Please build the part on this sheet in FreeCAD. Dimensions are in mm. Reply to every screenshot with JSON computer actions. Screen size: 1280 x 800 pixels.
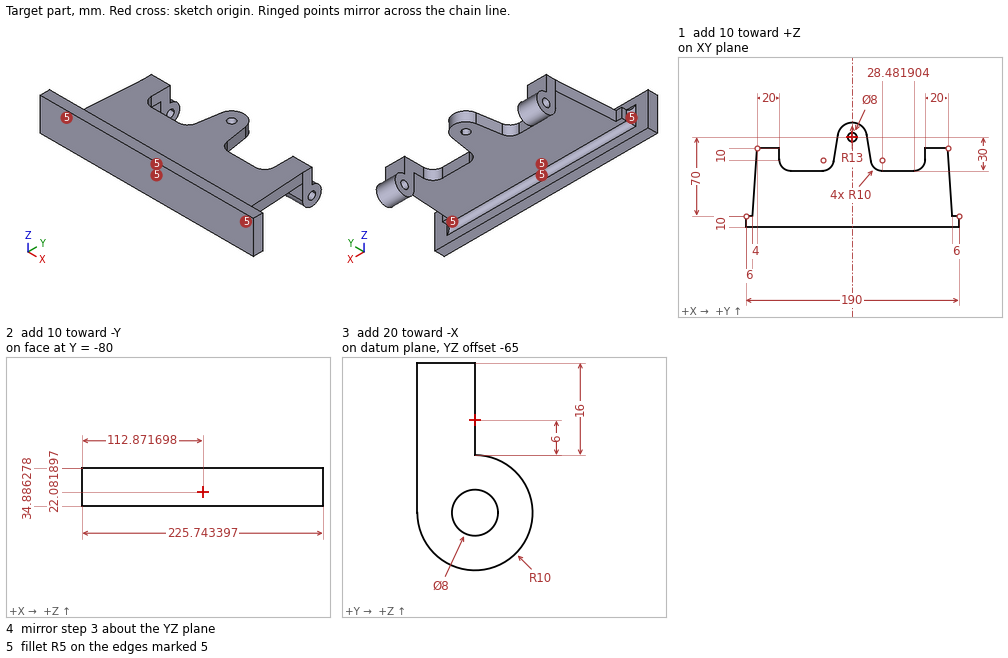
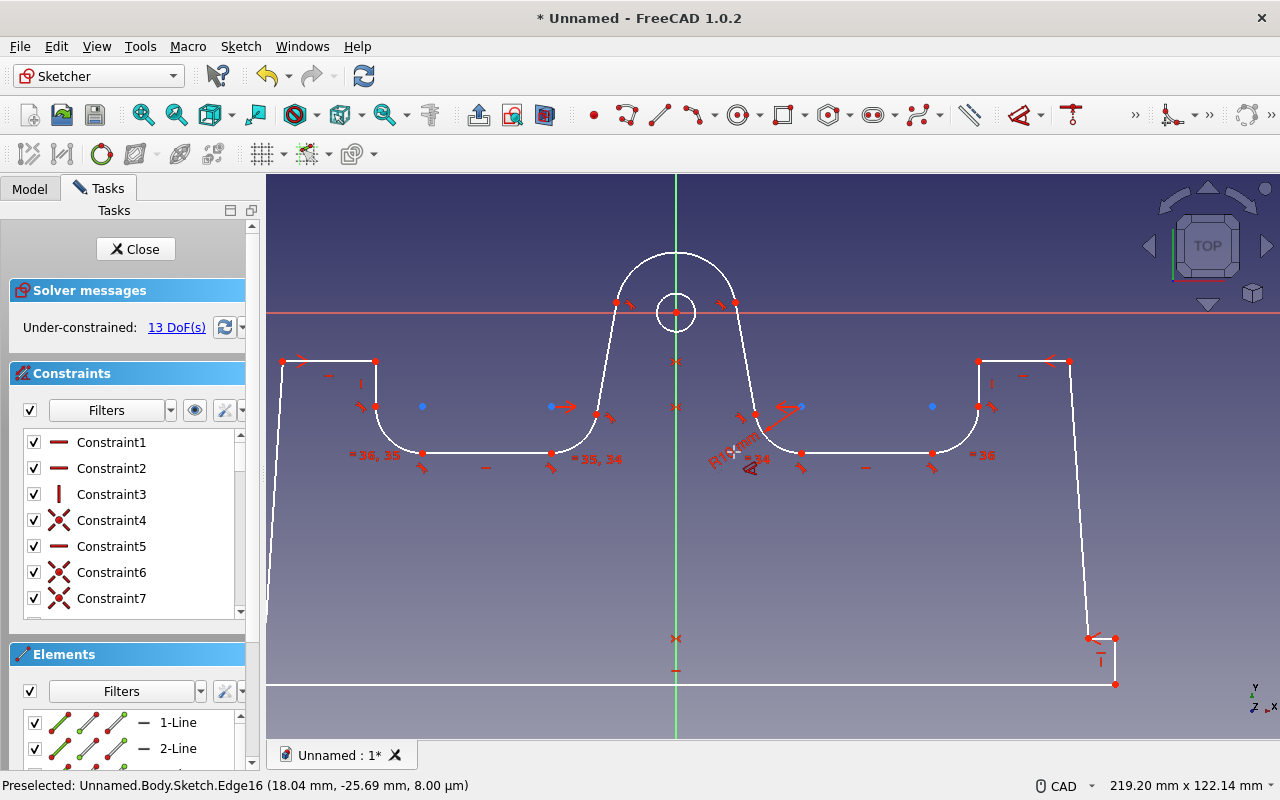
{"action": "left_click", "coordinate": [708, 262]}
{"action": "left_click", "coordinate": [725, 235]}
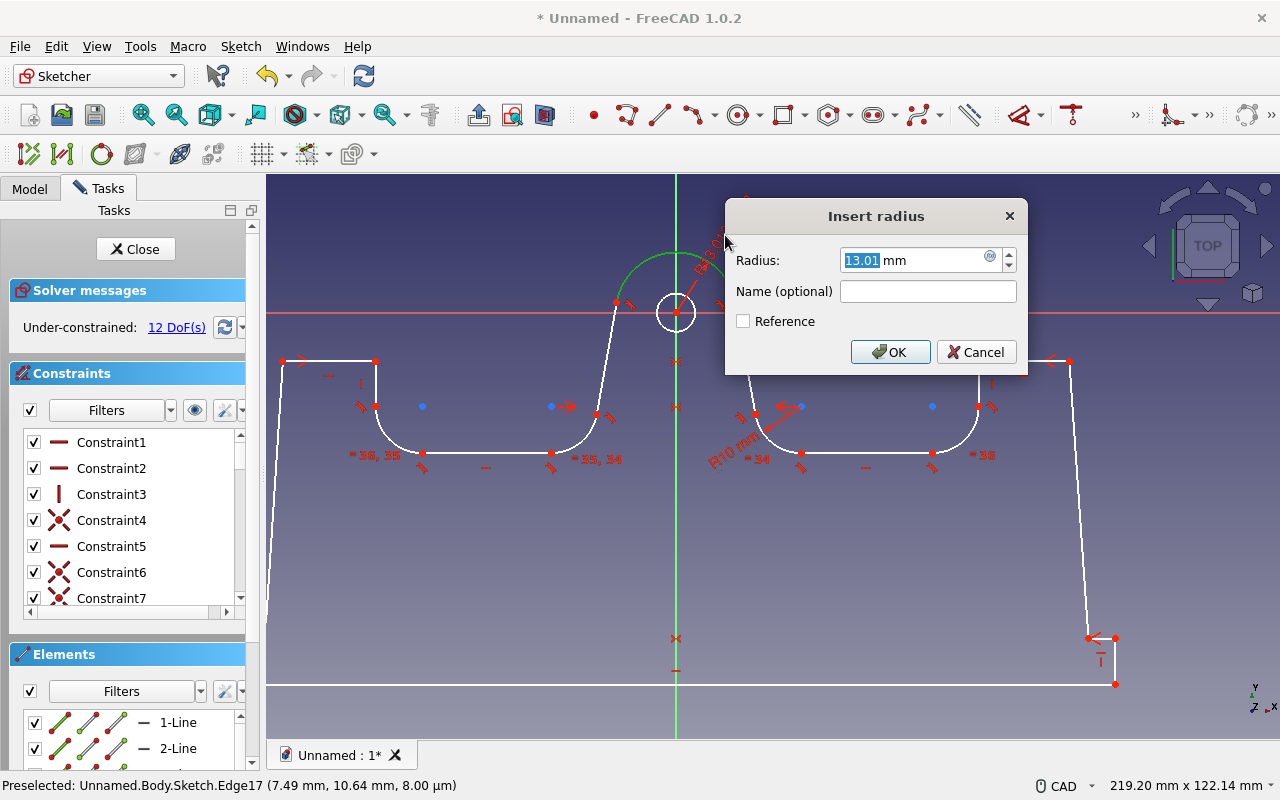
{"action": "type", "text": "13"}
{"action": "key", "text": "Return"}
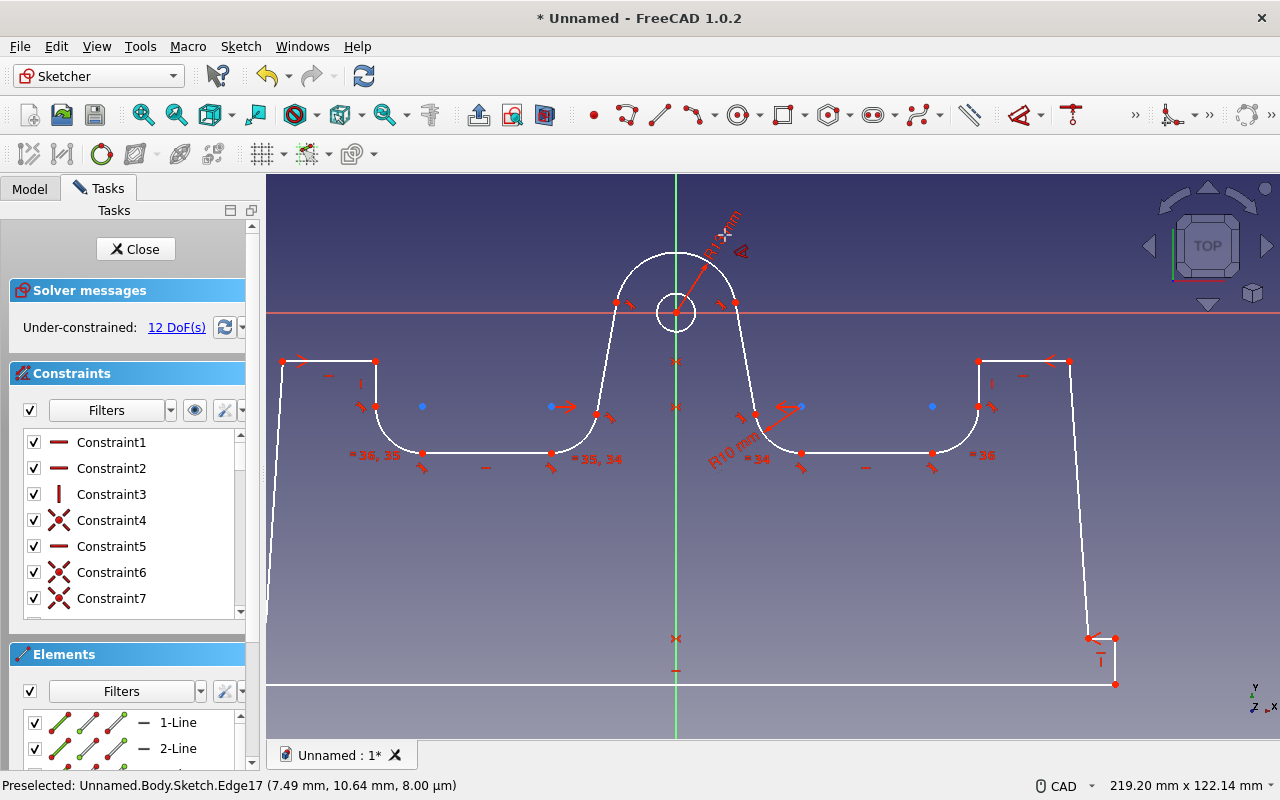
{"action": "left_click", "coordinate": [690, 299]}
{"action": "left_click", "coordinate": [712, 349]}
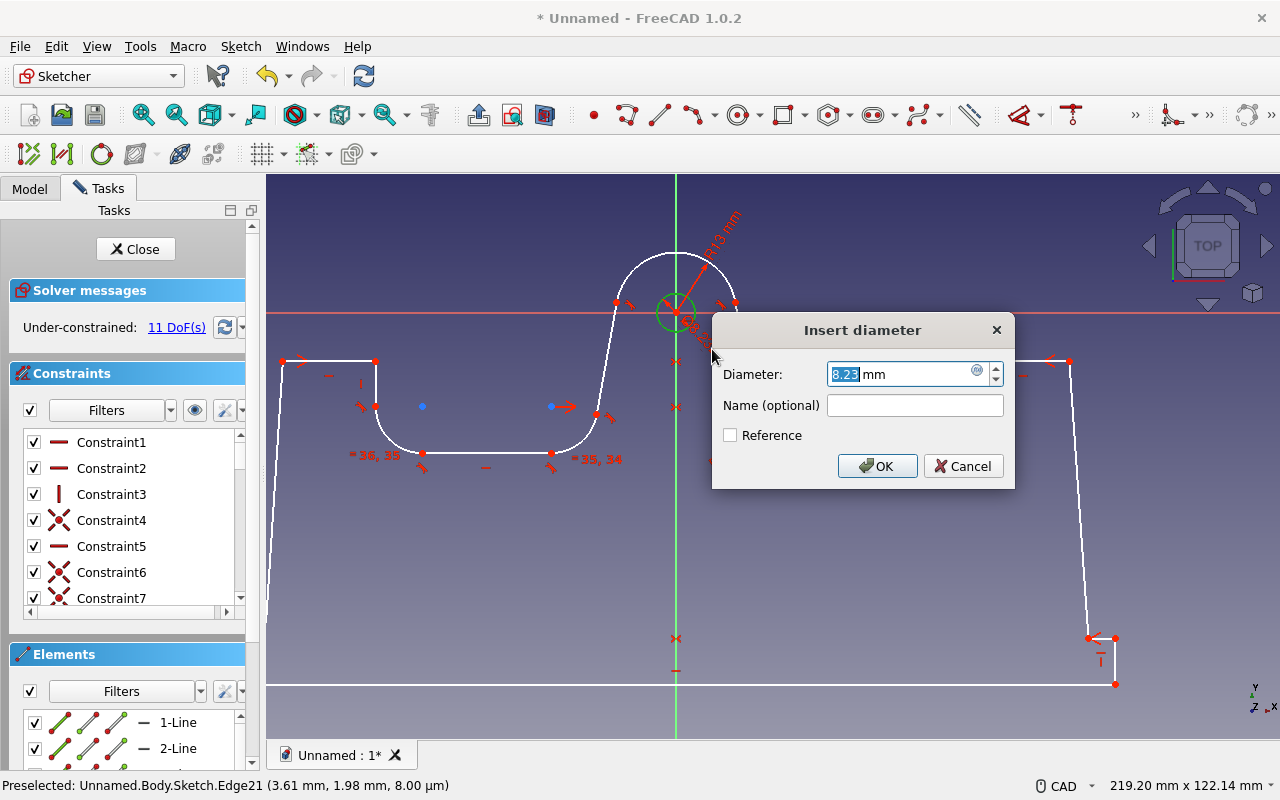
{"action": "type", "text": "8"}
{"action": "key", "text": "Return"}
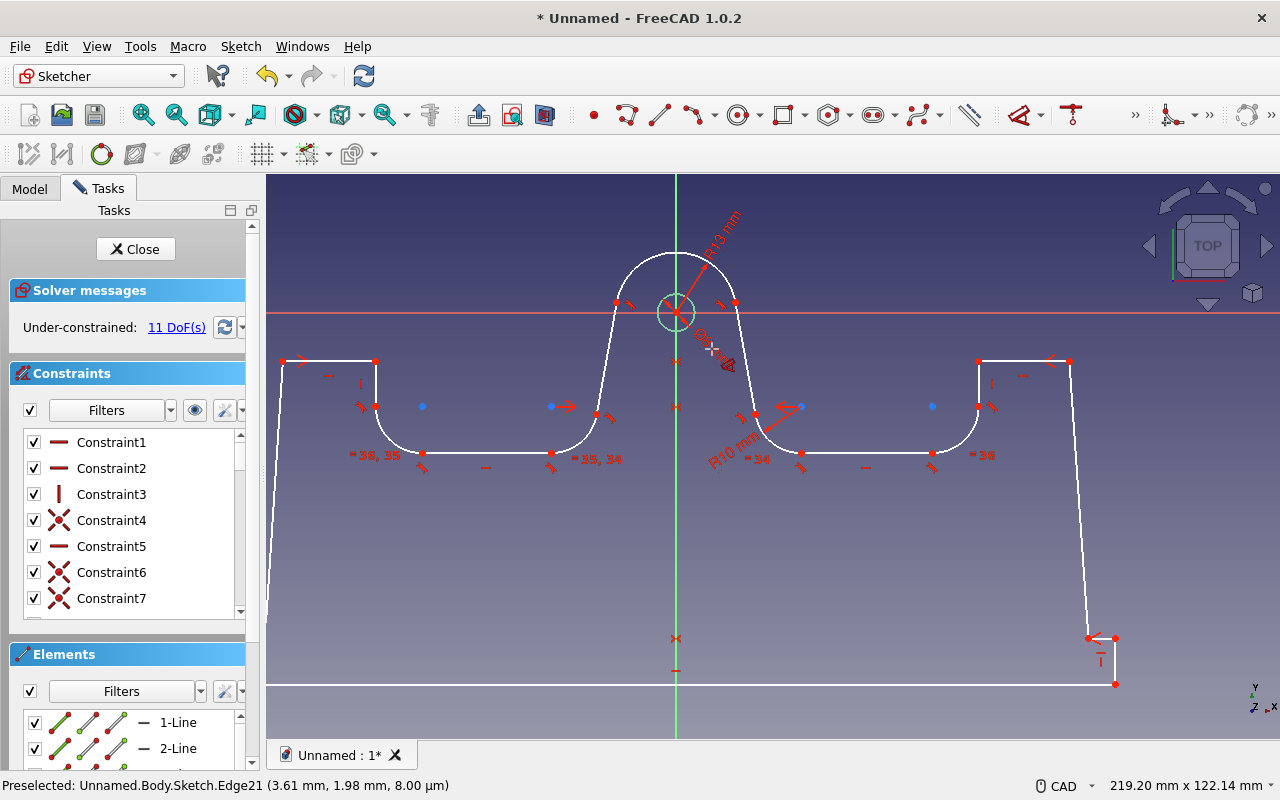
{"action": "scroll", "coordinate": [762, 434], "scroll_direction": "down", "scroll_amount": 2}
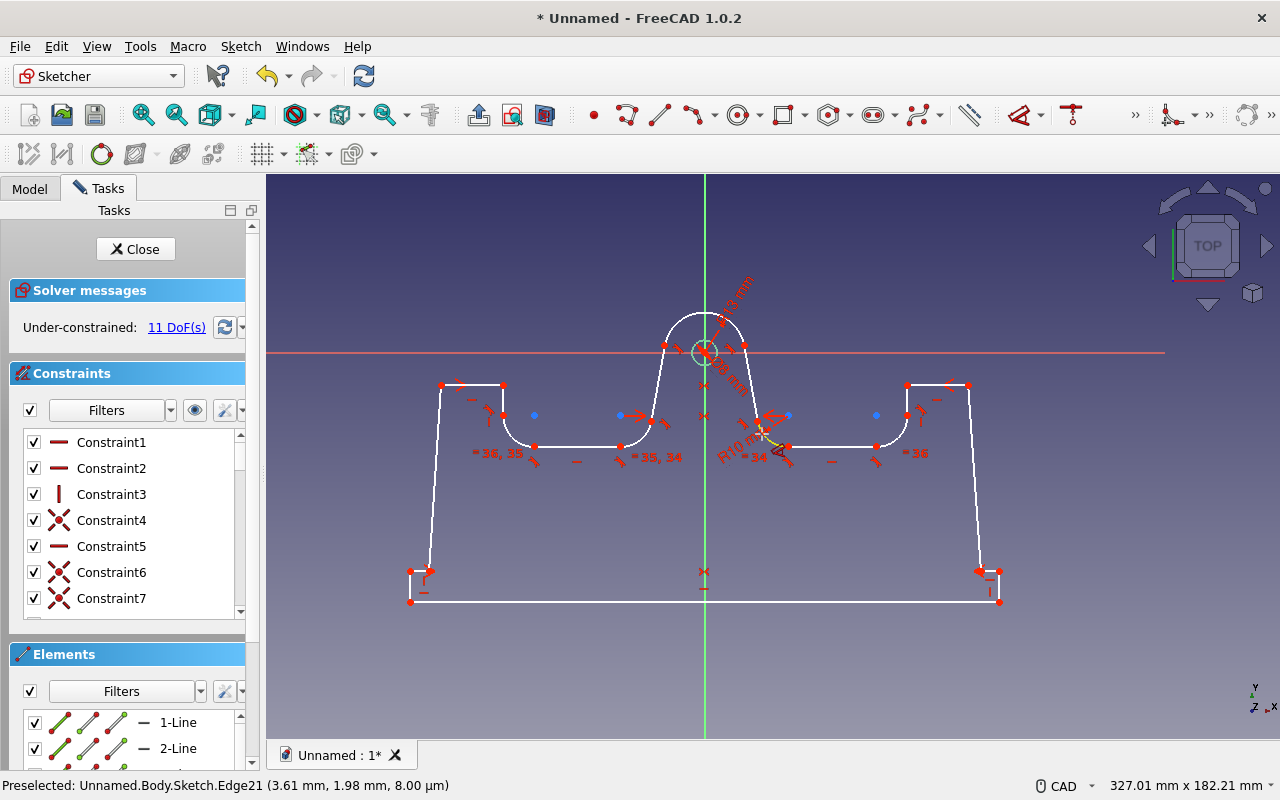
{"action": "scroll", "coordinate": [421, 571], "scroll_direction": "up", "scroll_amount": 4}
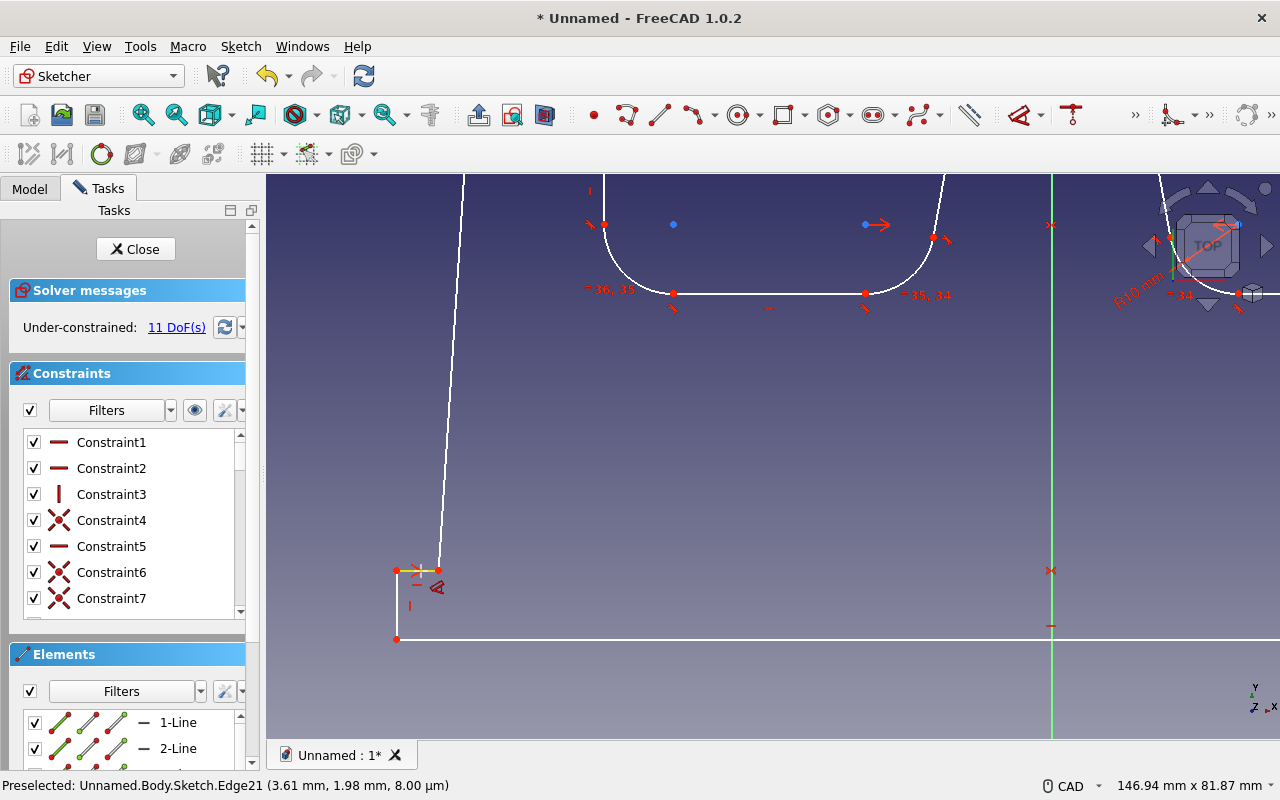
{"action": "left_click", "coordinate": [422, 571]}
{"action": "left_click", "coordinate": [418, 605]}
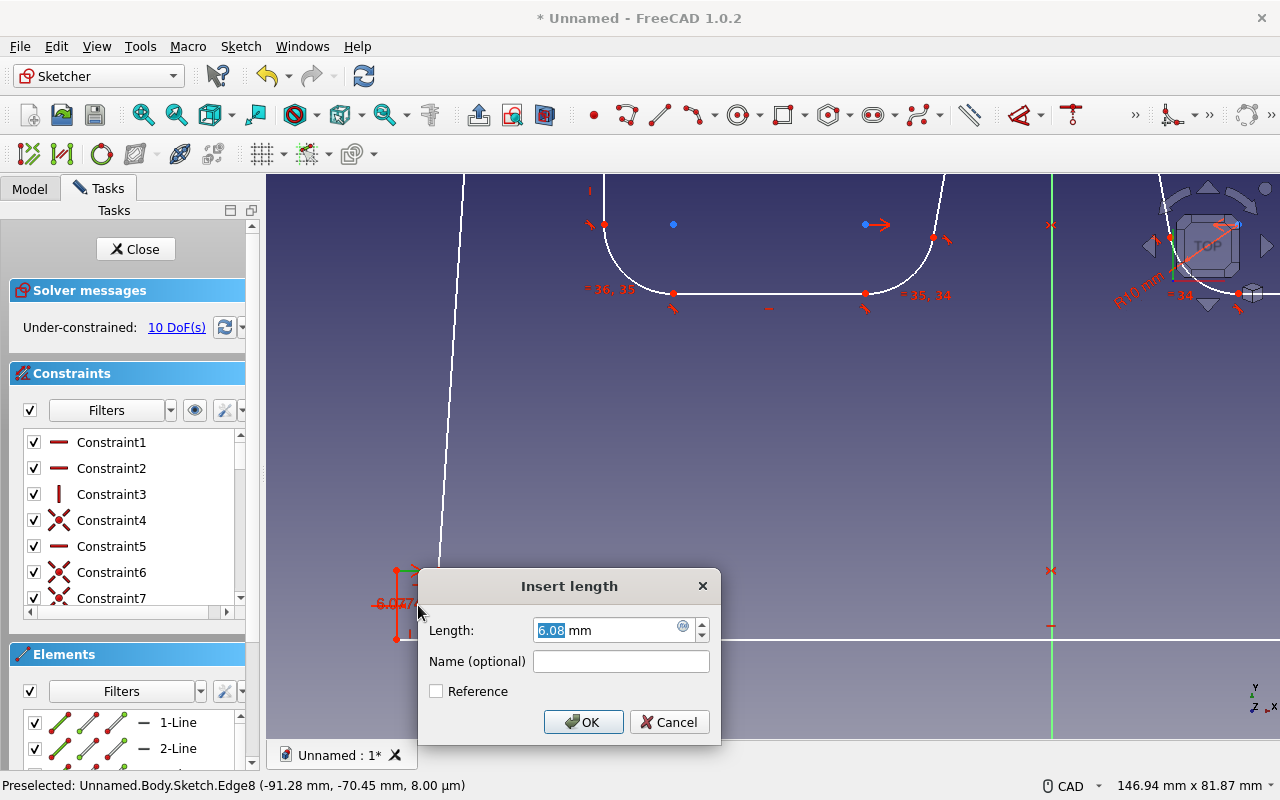
{"action": "type", "text": "6"}
{"action": "key", "text": "Return"}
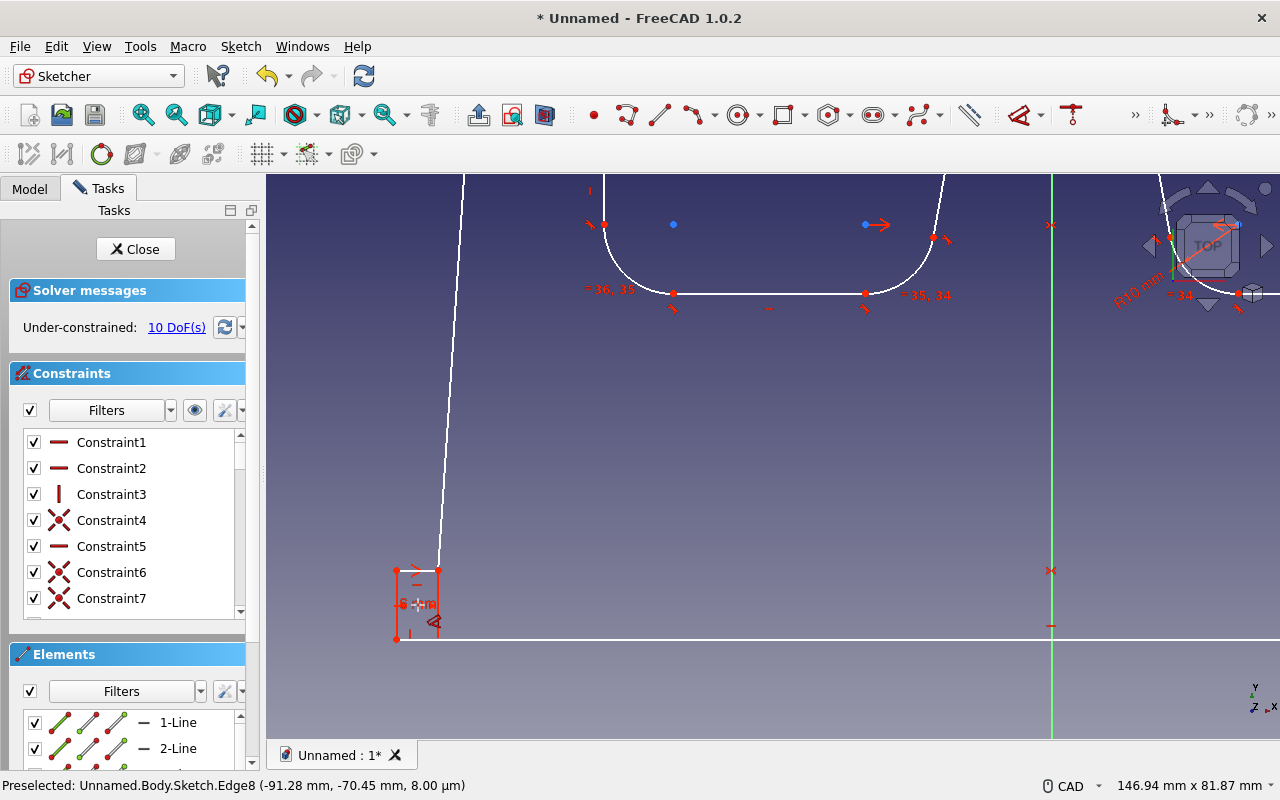
{"action": "scroll", "coordinate": [421, 571], "scroll_direction": "down", "scroll_amount": 4}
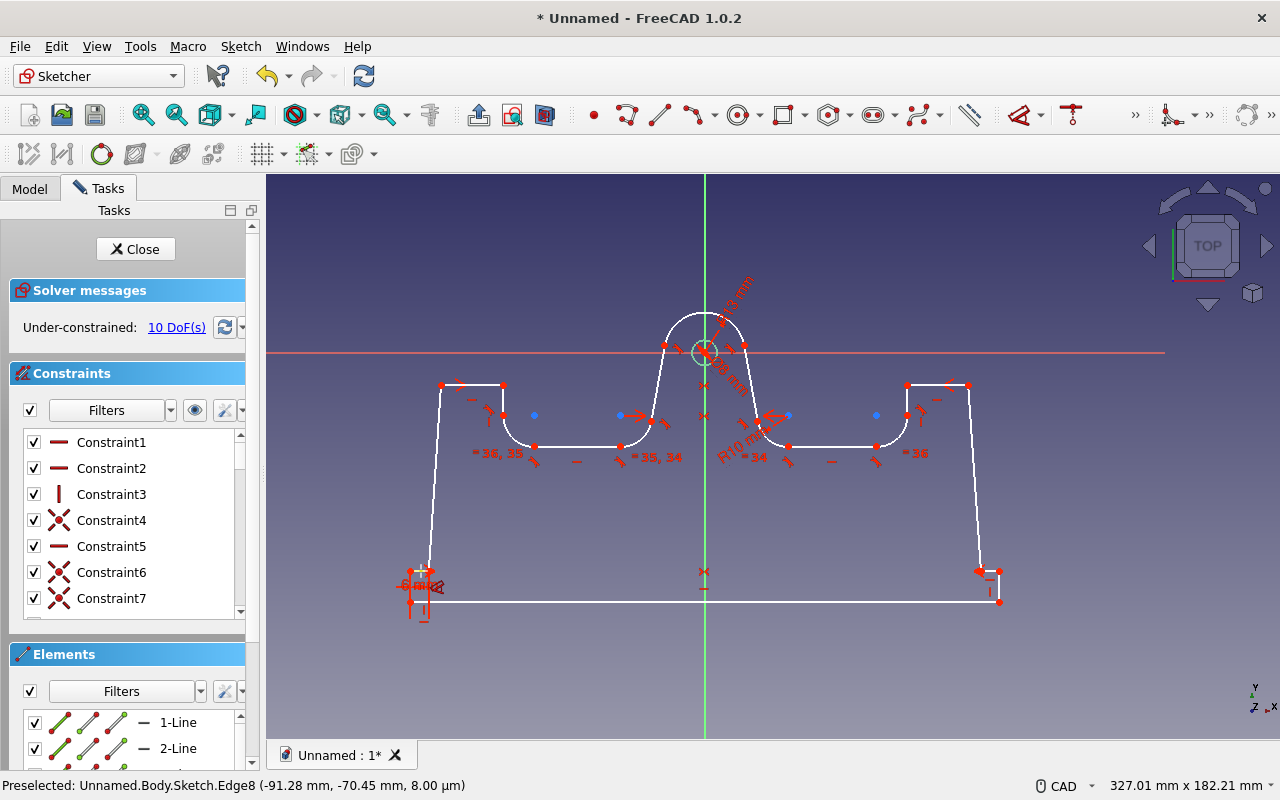
{"action": "scroll", "coordinate": [994, 571], "scroll_direction": "up", "scroll_amount": 5}